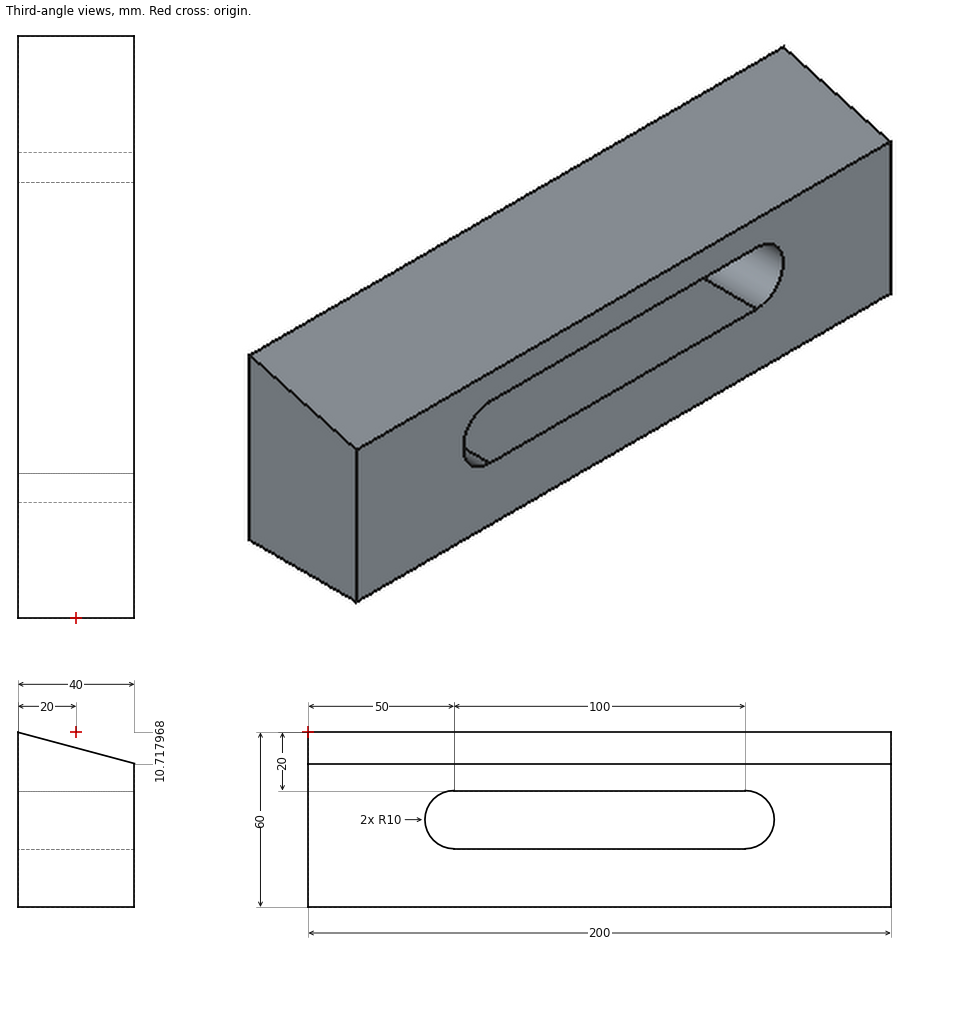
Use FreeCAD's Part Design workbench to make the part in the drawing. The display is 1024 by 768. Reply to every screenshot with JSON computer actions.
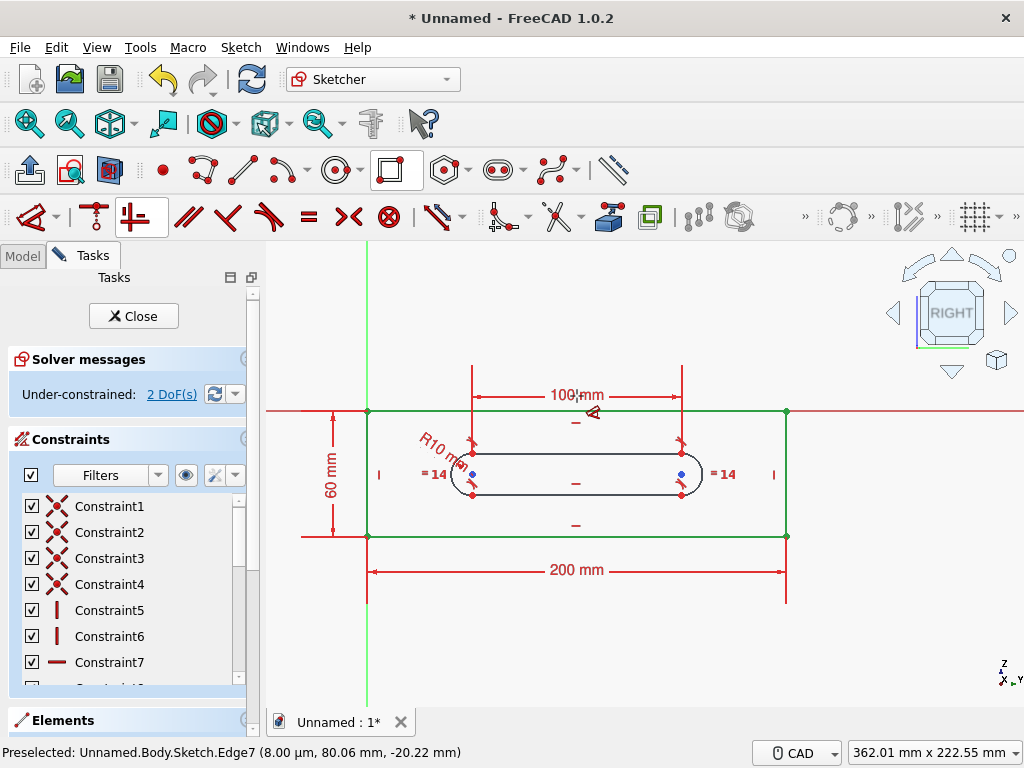
{"action": "left_click", "coordinate": [472, 454]}
{"action": "left_click", "coordinate": [420, 377]}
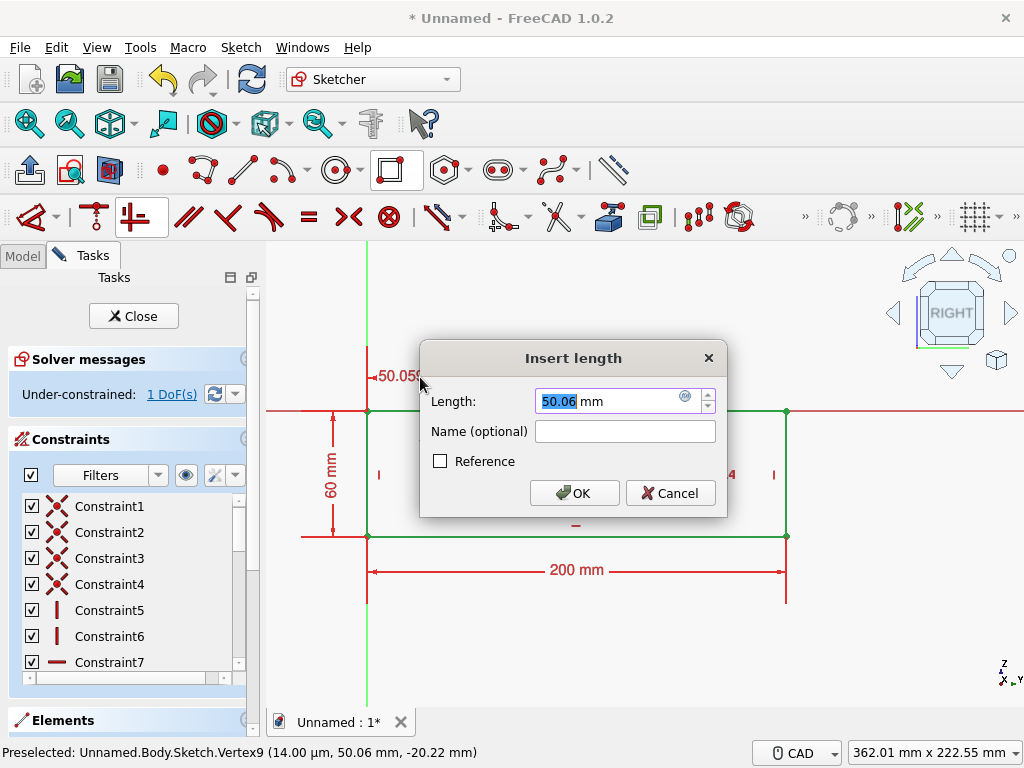
{"action": "type", "text": "50"}
{"action": "key", "text": "Return"}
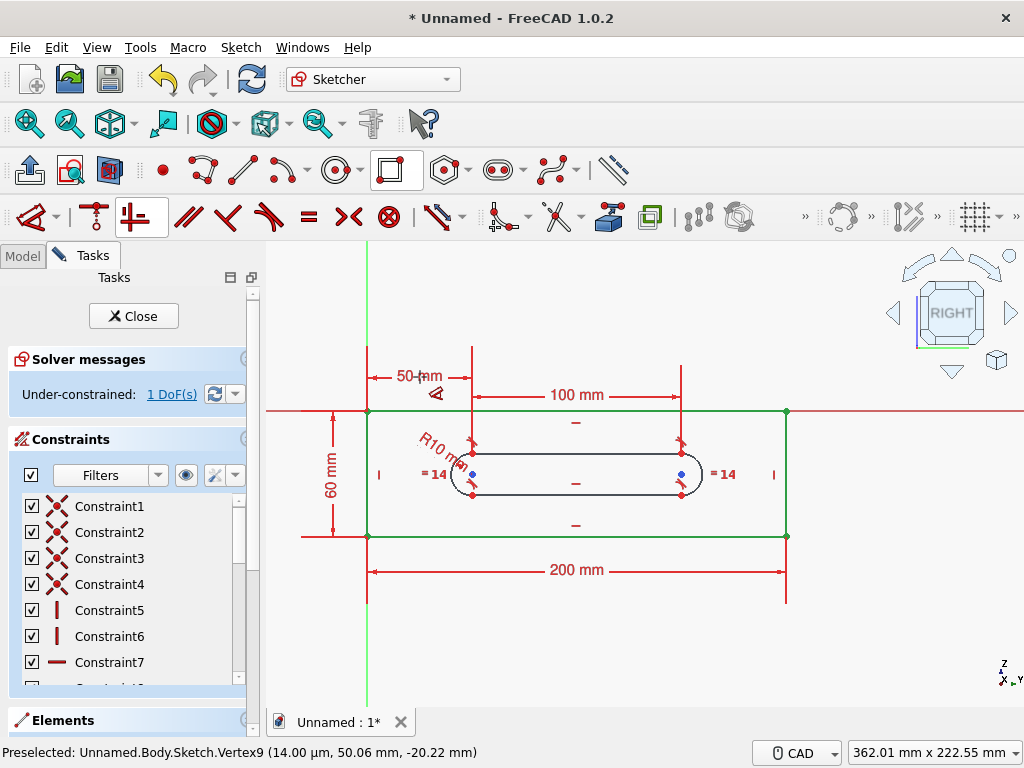
{"action": "left_click", "coordinate": [472, 454]}
{"action": "left_click", "coordinate": [333, 432]}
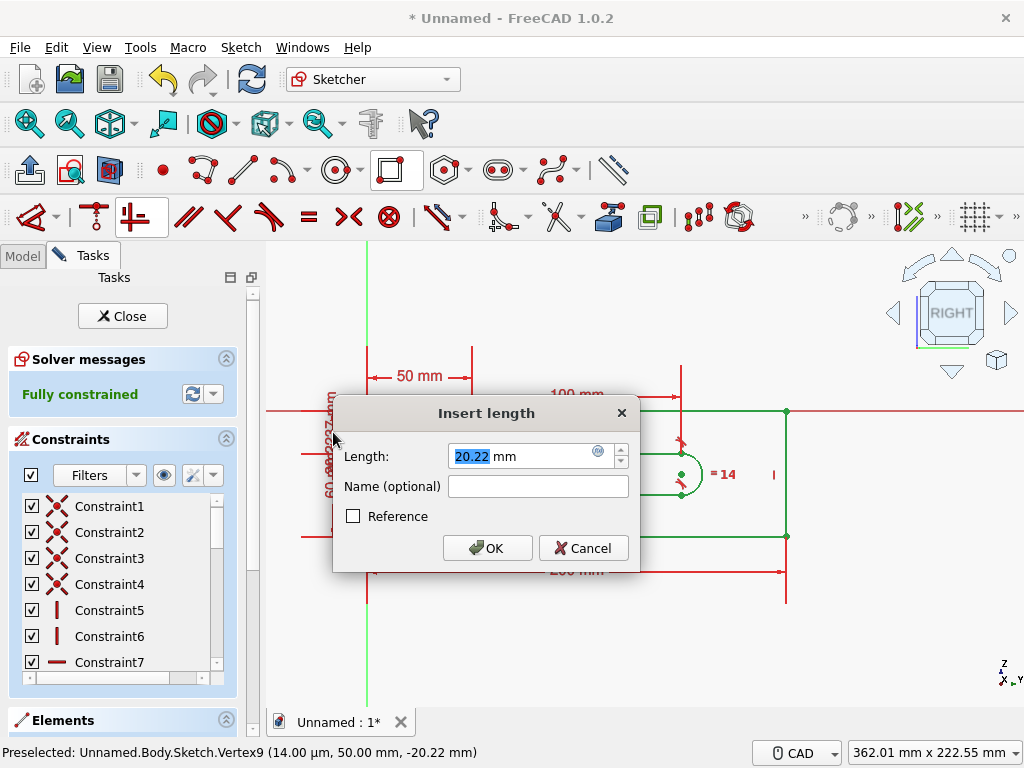
{"action": "type", "text": "20"}
{"action": "key", "text": "Return"}
{"action": "key", "text": "Escape"}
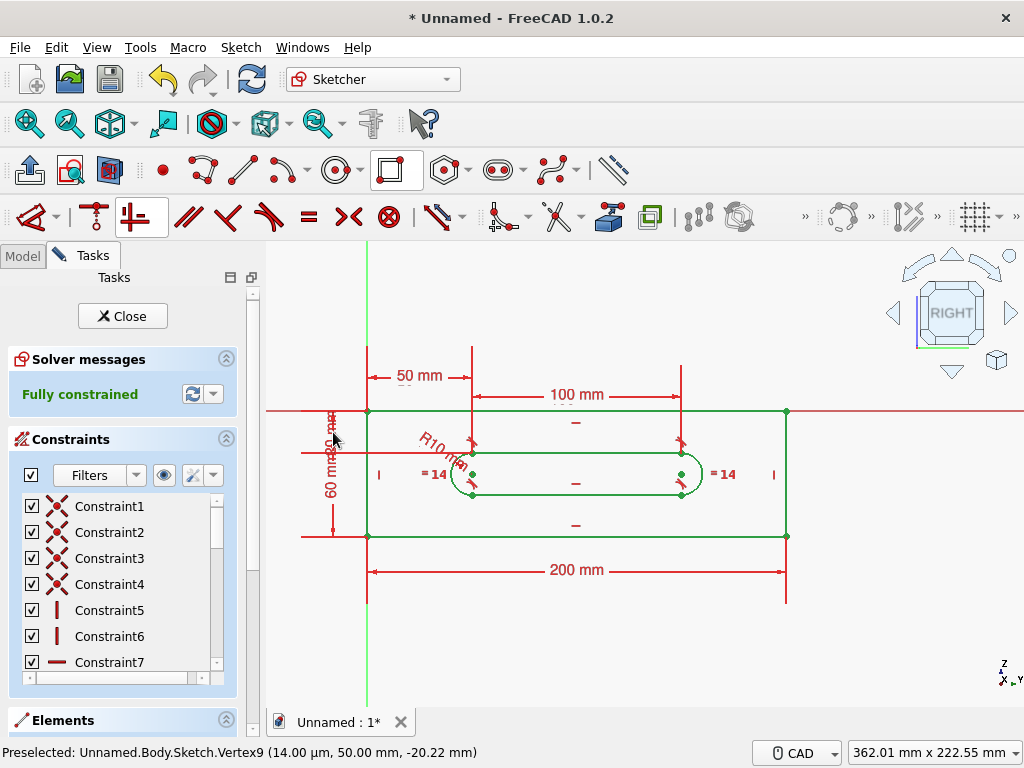
{"action": "left_click", "coordinate": [123, 316]}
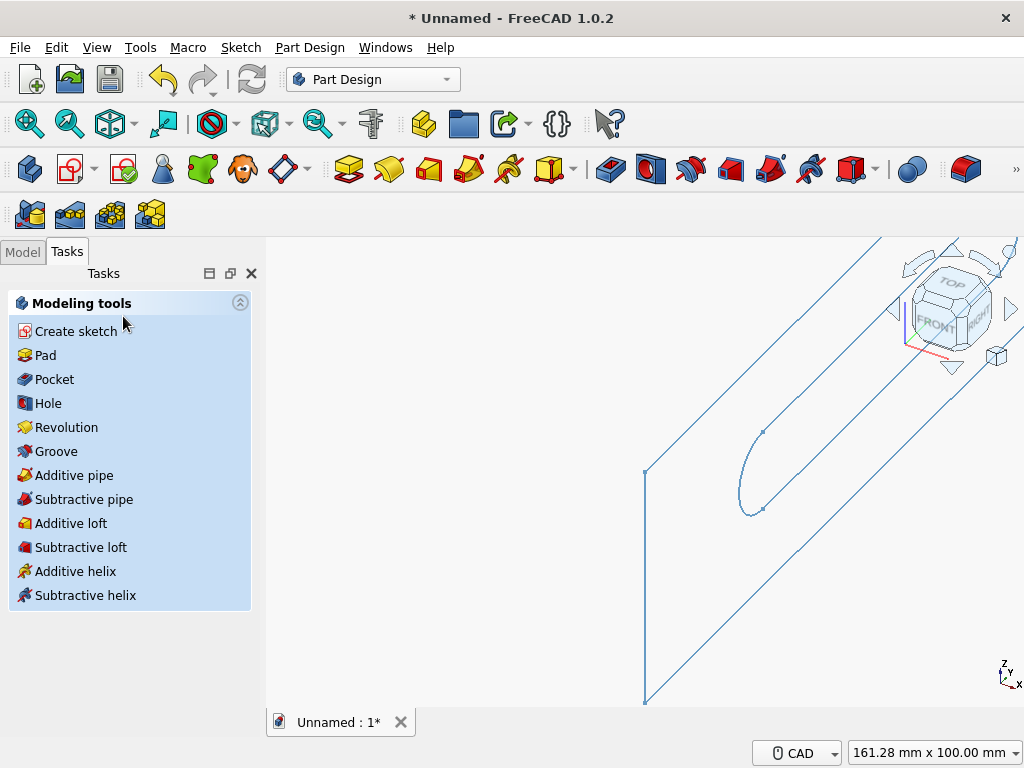
{"action": "left_click", "coordinate": [350, 170]}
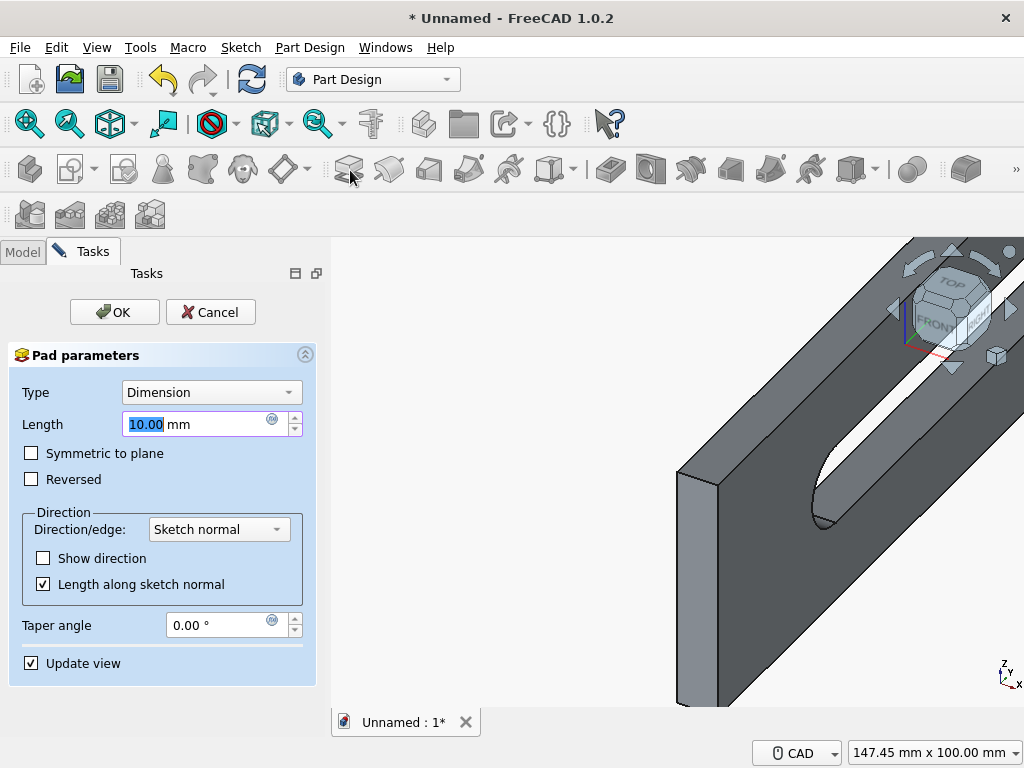
{"action": "type", "text": "40"}
{"action": "key", "text": "Tab"}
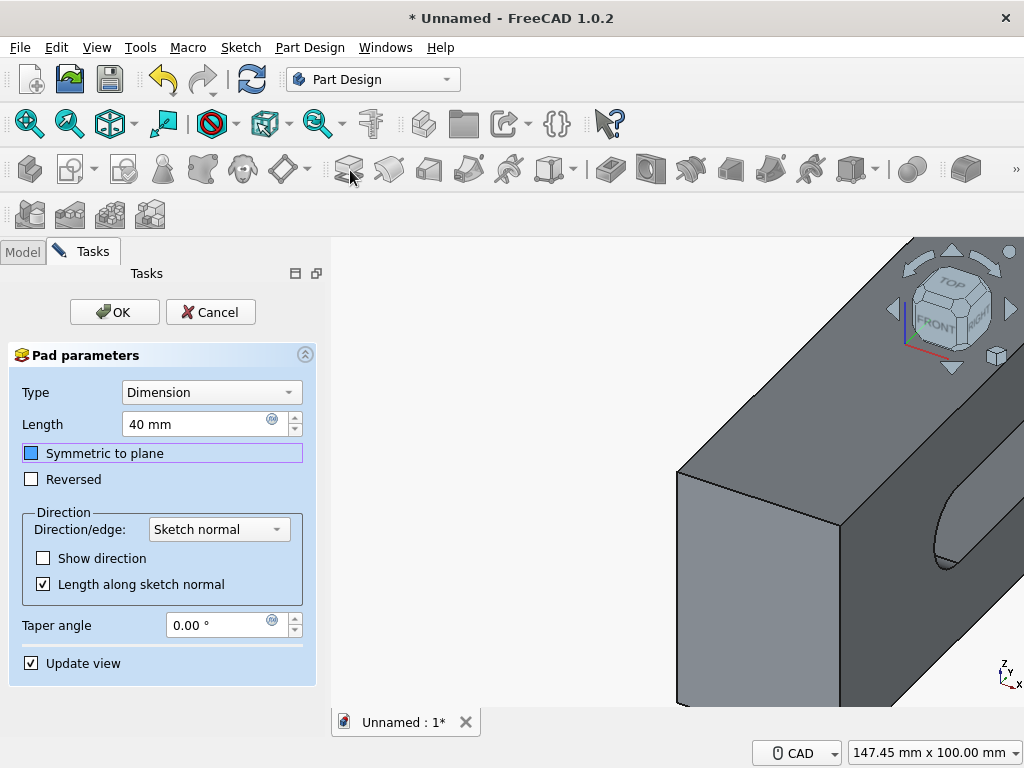
{"action": "left_click", "coordinate": [30, 453]}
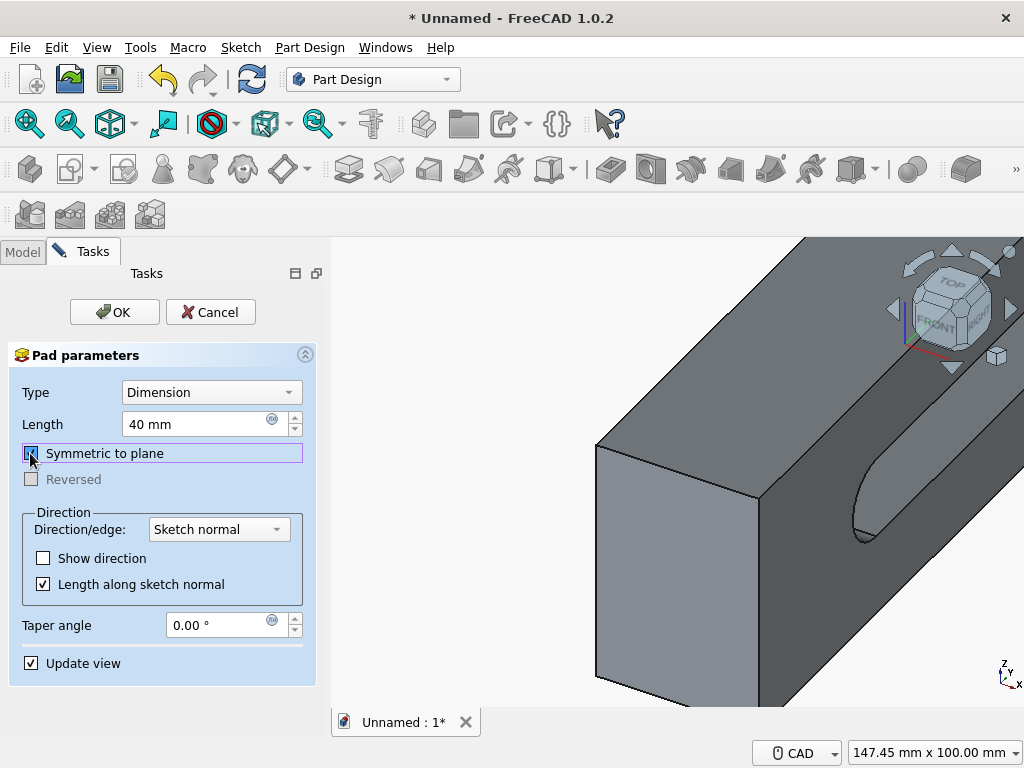
{"action": "left_click", "coordinate": [115, 312]}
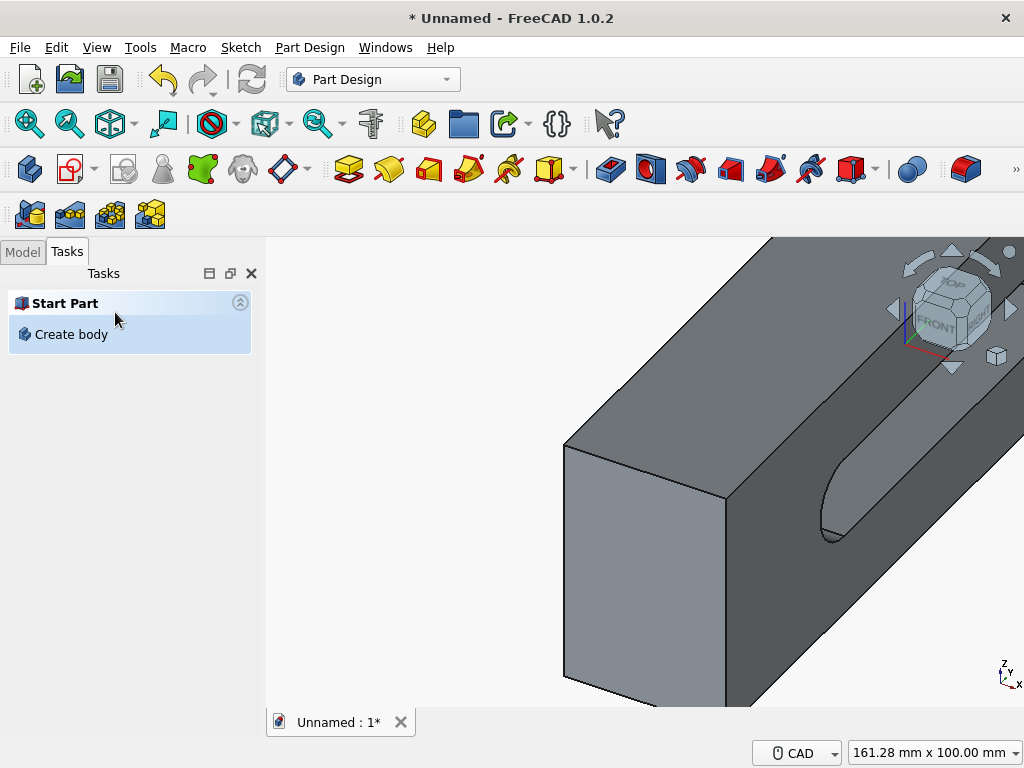
{"action": "left_click", "coordinate": [30, 124]}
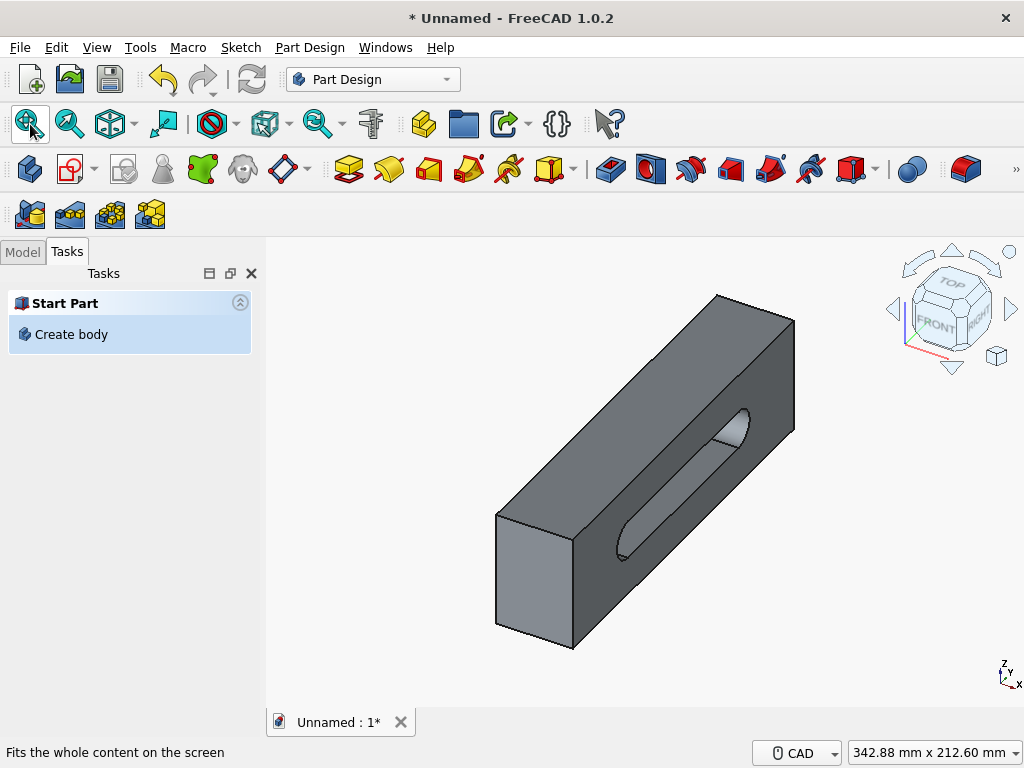
{"action": "left_click", "coordinate": [534, 581]}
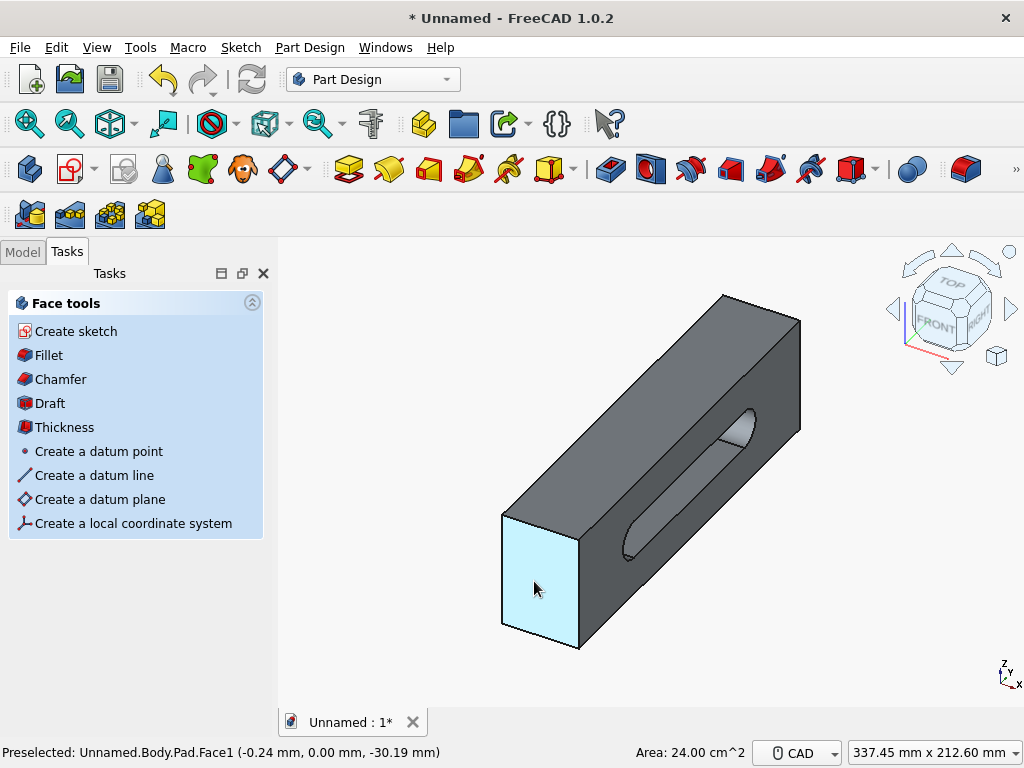
{"action": "left_click", "coordinate": [70, 170]}